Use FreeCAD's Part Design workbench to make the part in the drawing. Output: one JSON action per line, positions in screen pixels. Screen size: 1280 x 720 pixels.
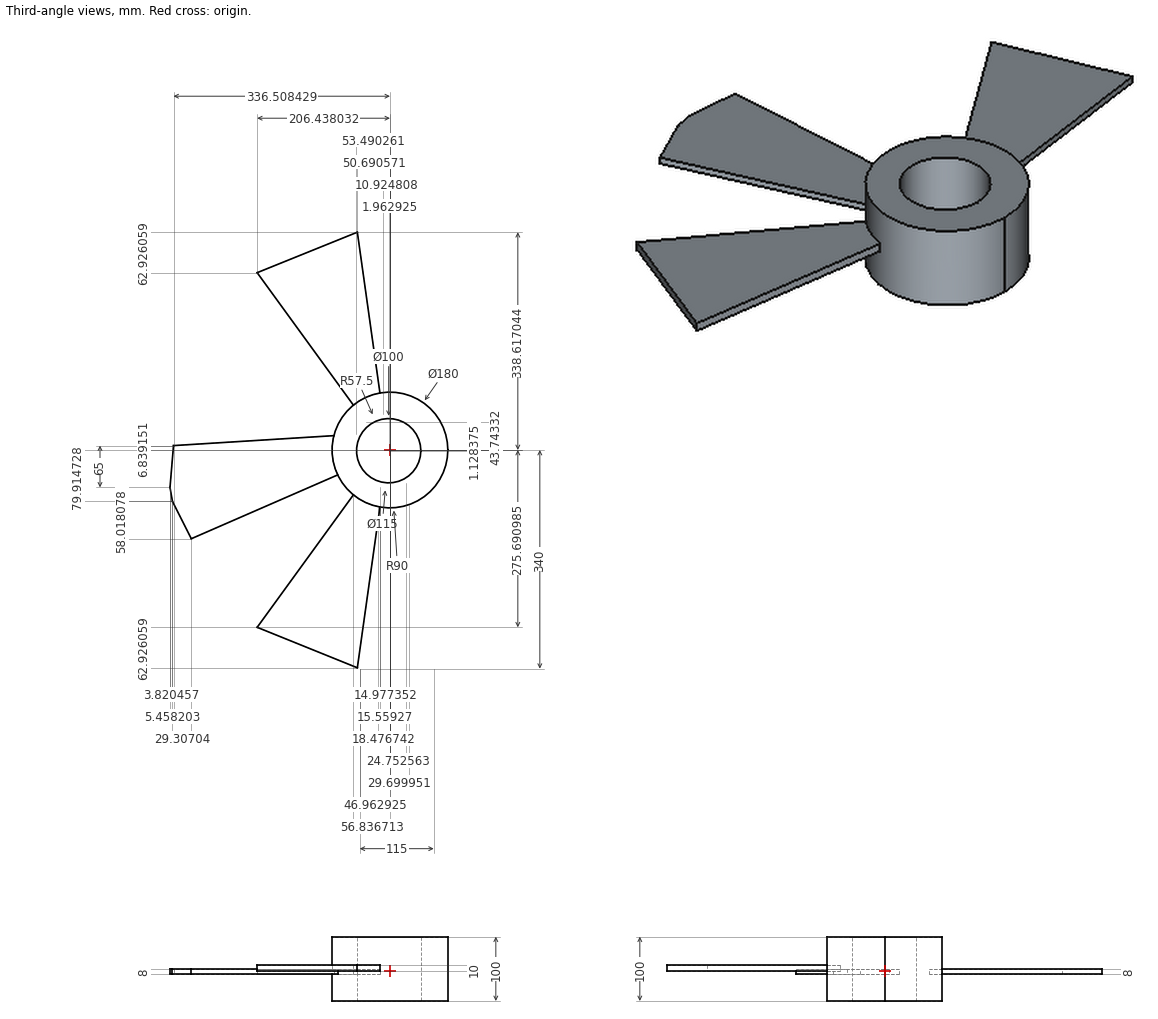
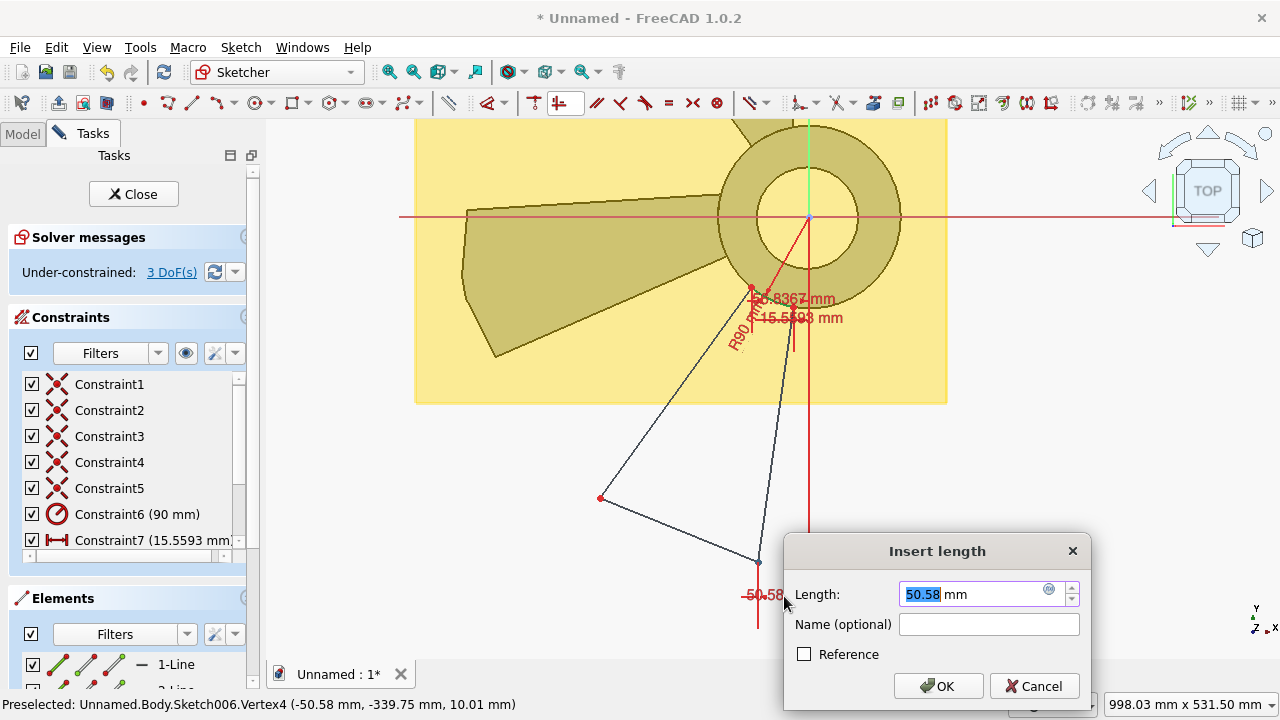
{"action": "type", "text": "50.690571"}
{"action": "key", "text": "Return"}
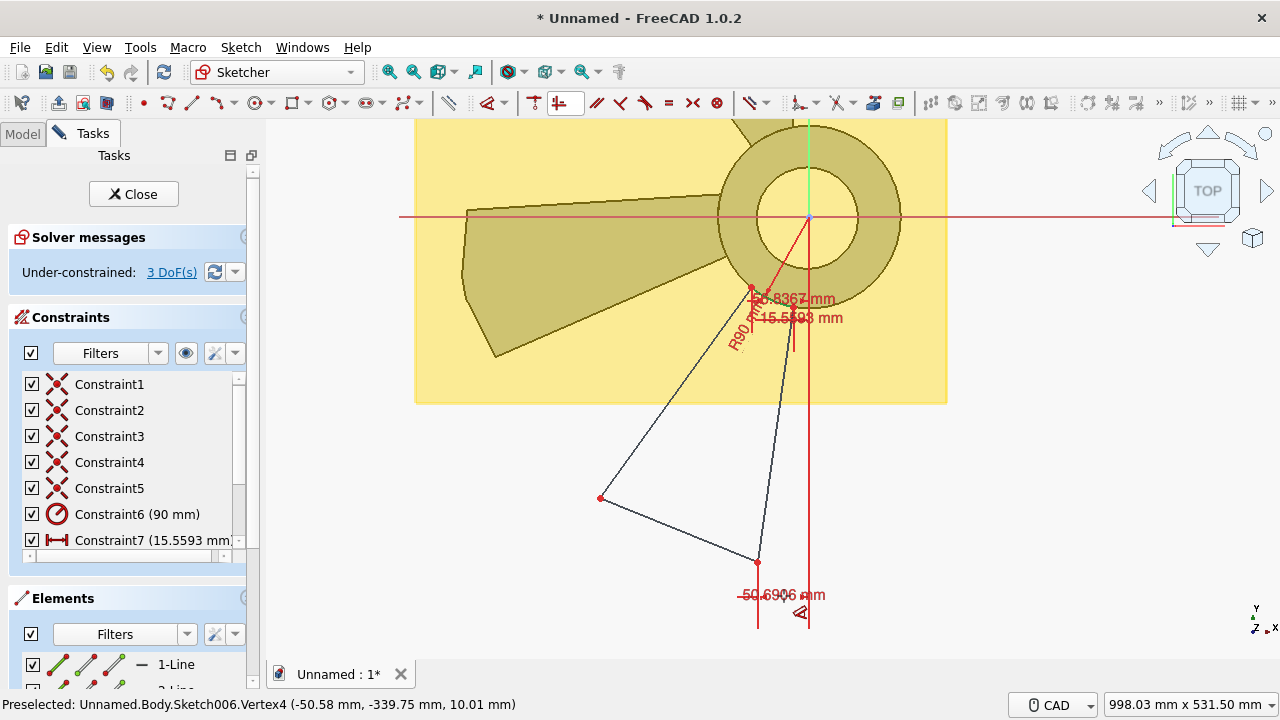
{"action": "left_click", "coordinate": [647, 517]}
{"action": "left_click", "coordinate": [566, 530]}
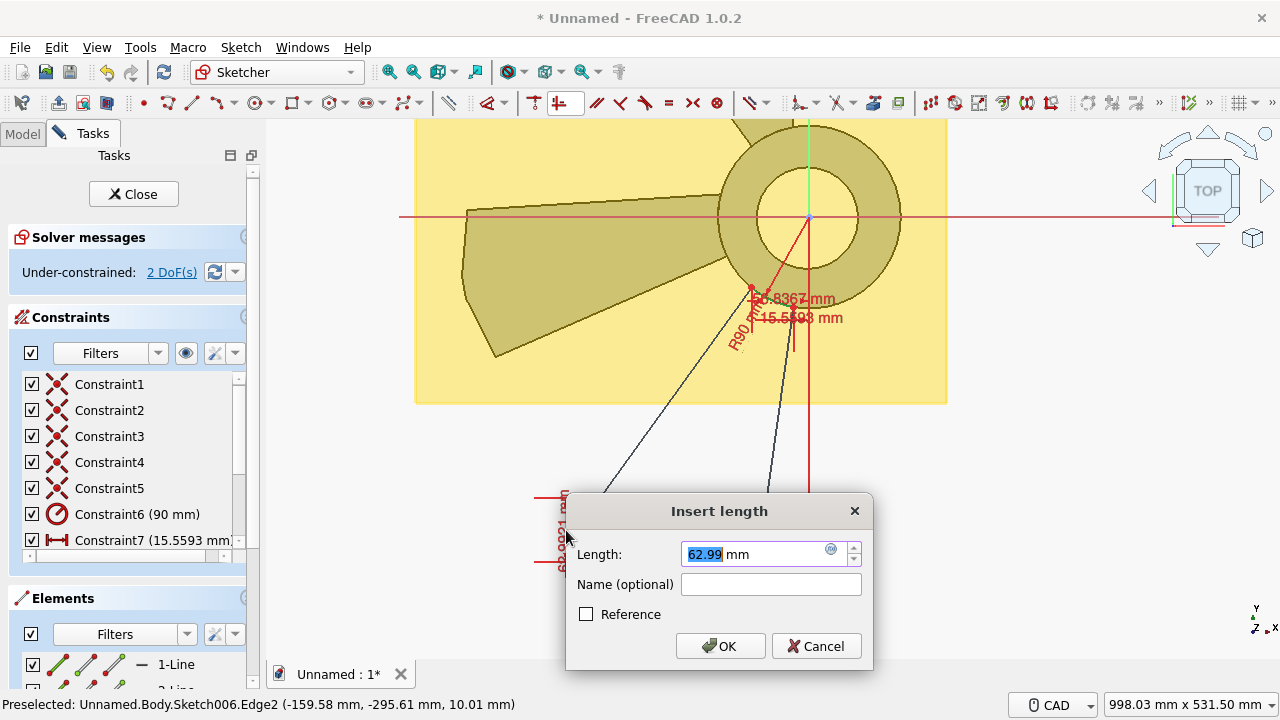
{"action": "type", "text": "62.926059"}
{"action": "key", "text": "Return"}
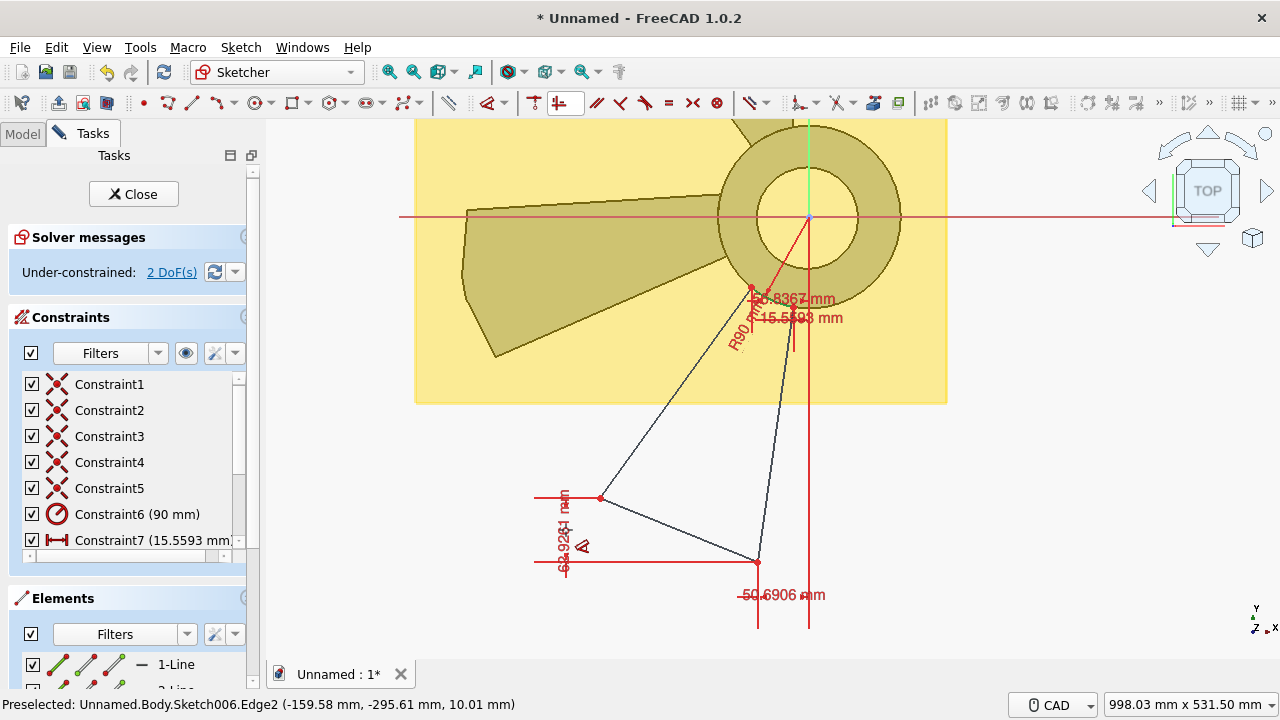
{"action": "left_click", "coordinate": [600, 498]}
{"action": "left_click", "coordinate": [705, 183]}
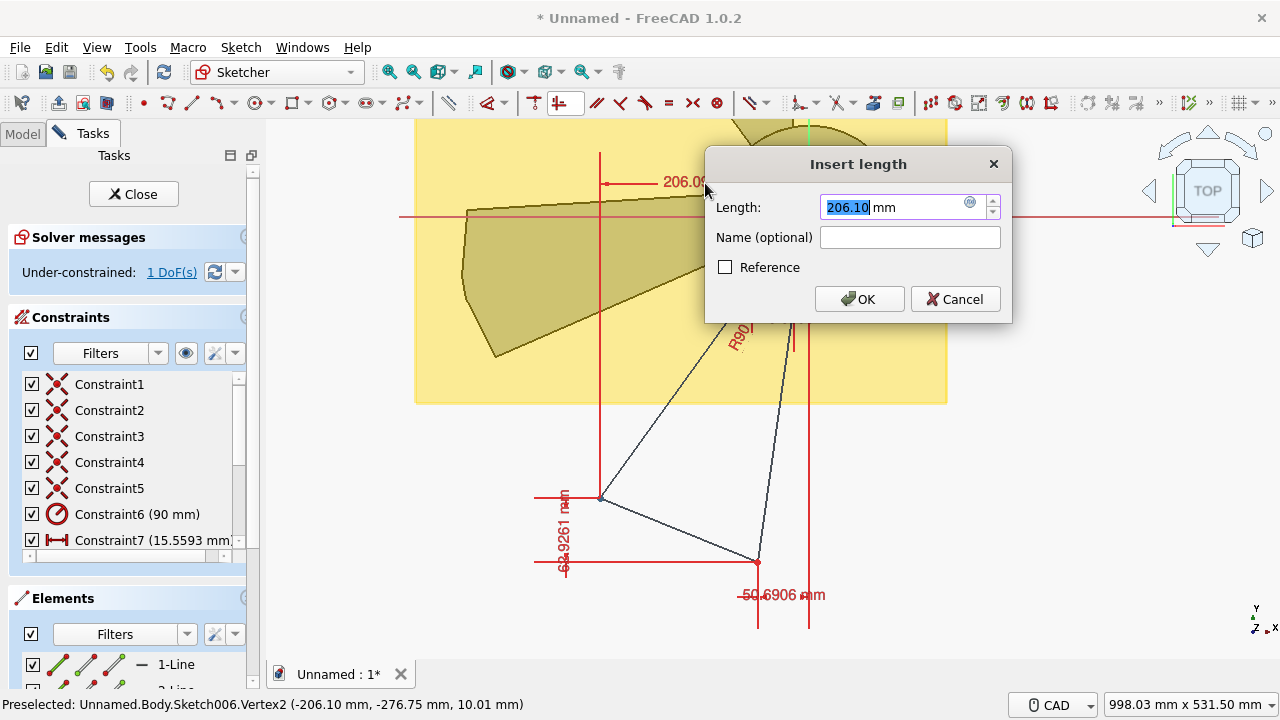
{"action": "type", "text": "206.438032"}
{"action": "key", "text": "Return"}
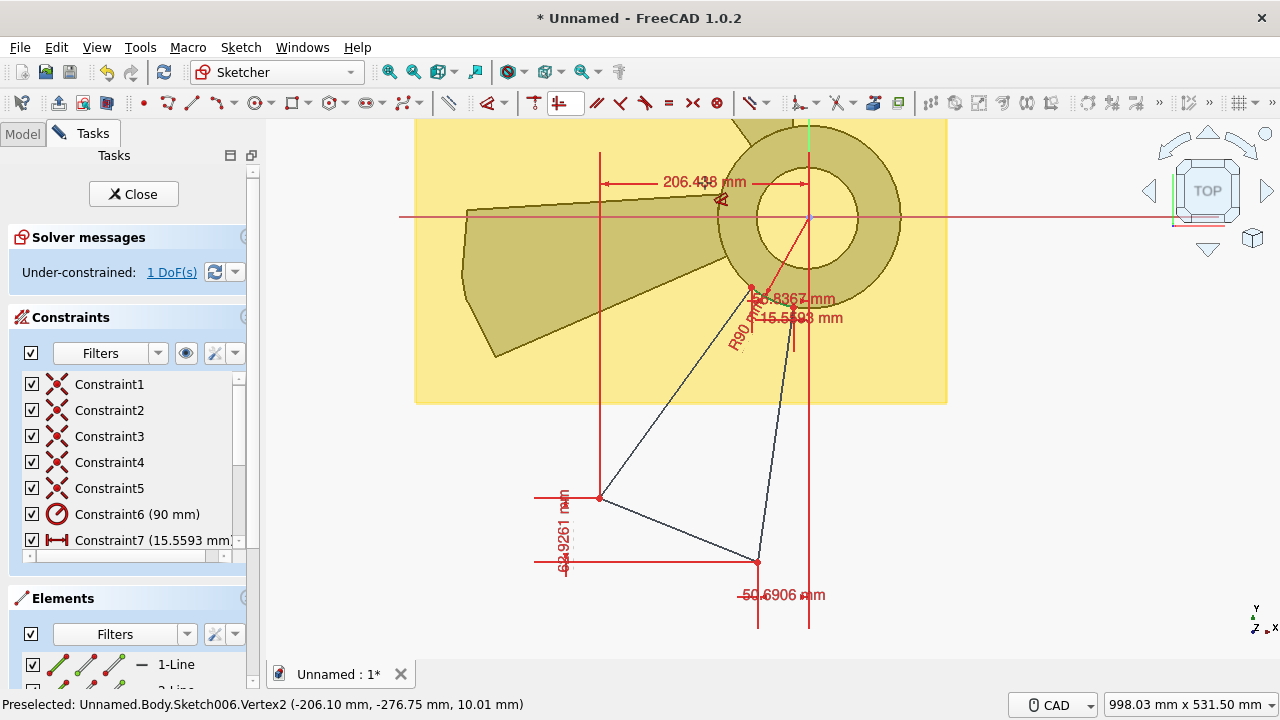
{"action": "left_click", "coordinate": [600, 498]}
{"action": "left_click", "coordinate": [566, 358]}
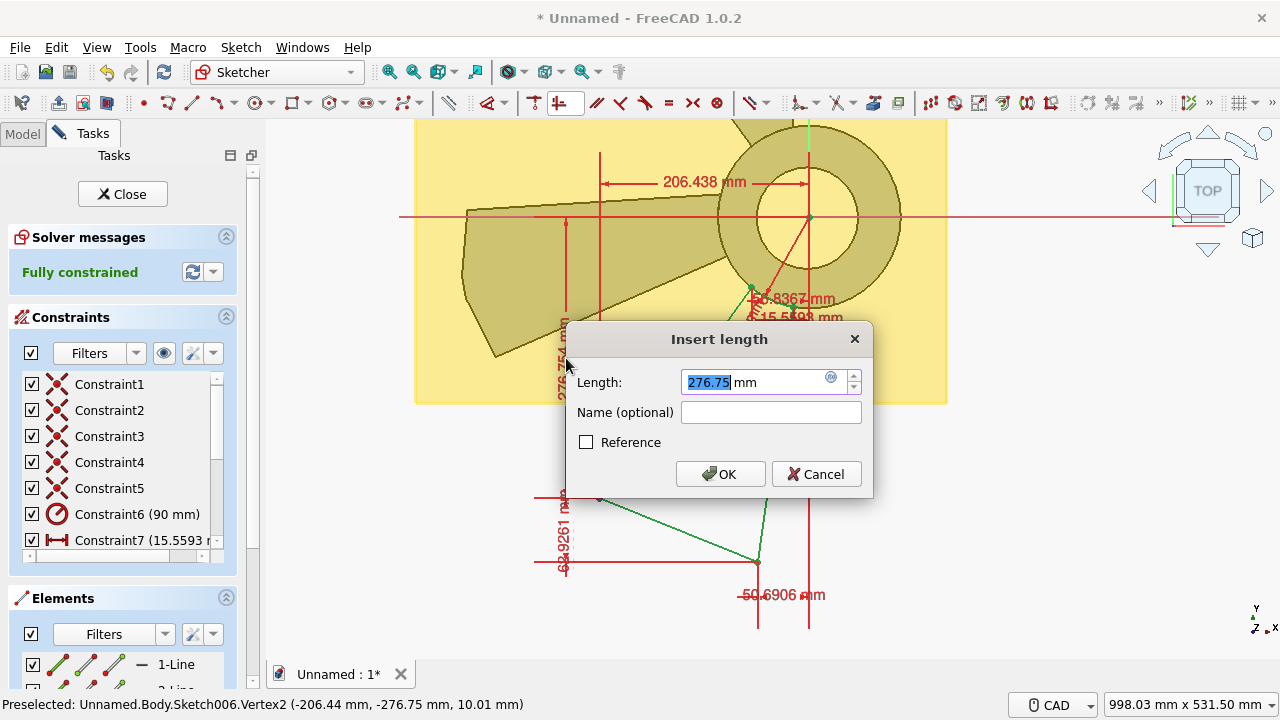
{"action": "type", "text": "275.690985"}
{"action": "key", "text": "Return"}
{"action": "key", "text": "Escape"}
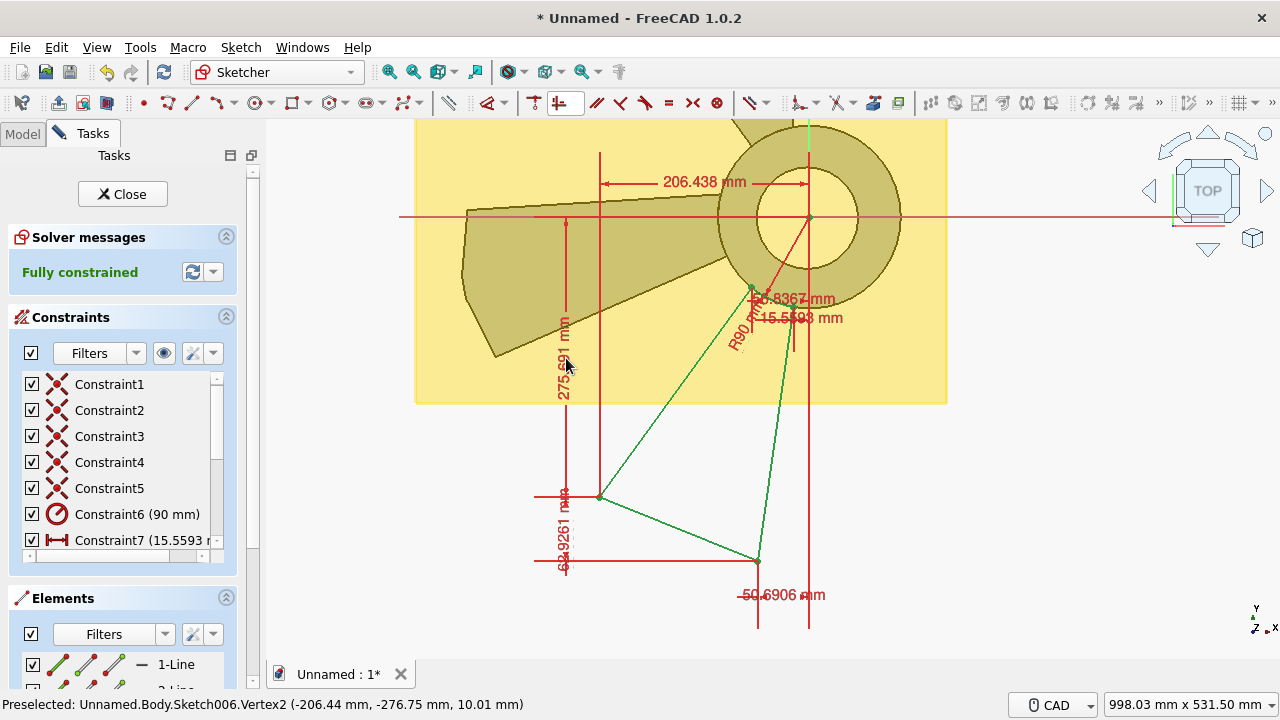
{"action": "left_click", "coordinate": [123, 194]}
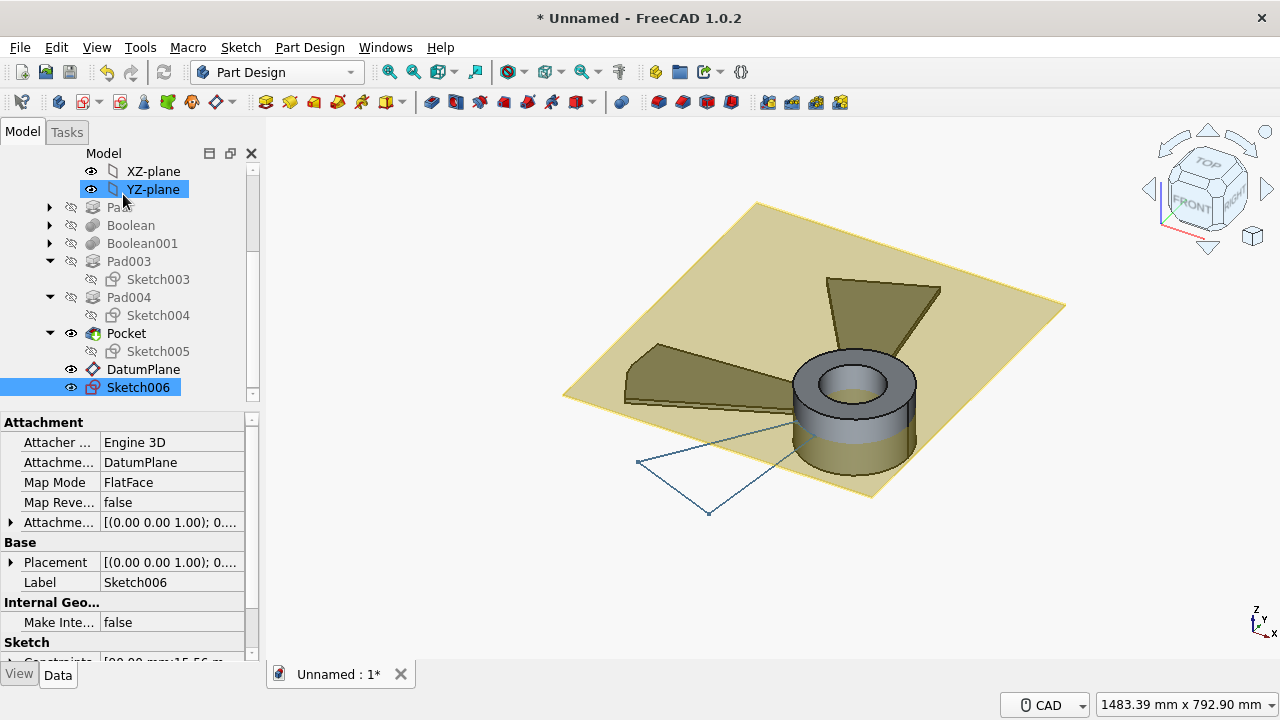
{"action": "left_click", "coordinate": [266, 102]}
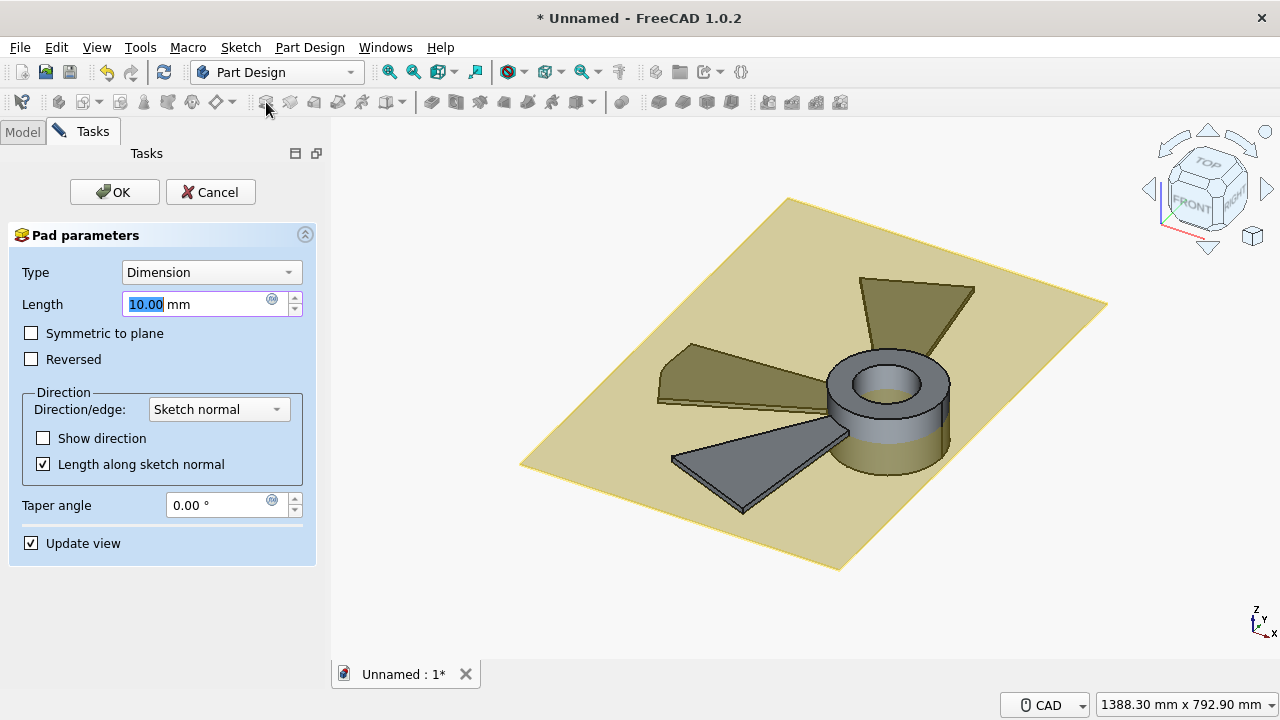
{"action": "type", "text": "10"}
{"action": "key", "text": "Tab"}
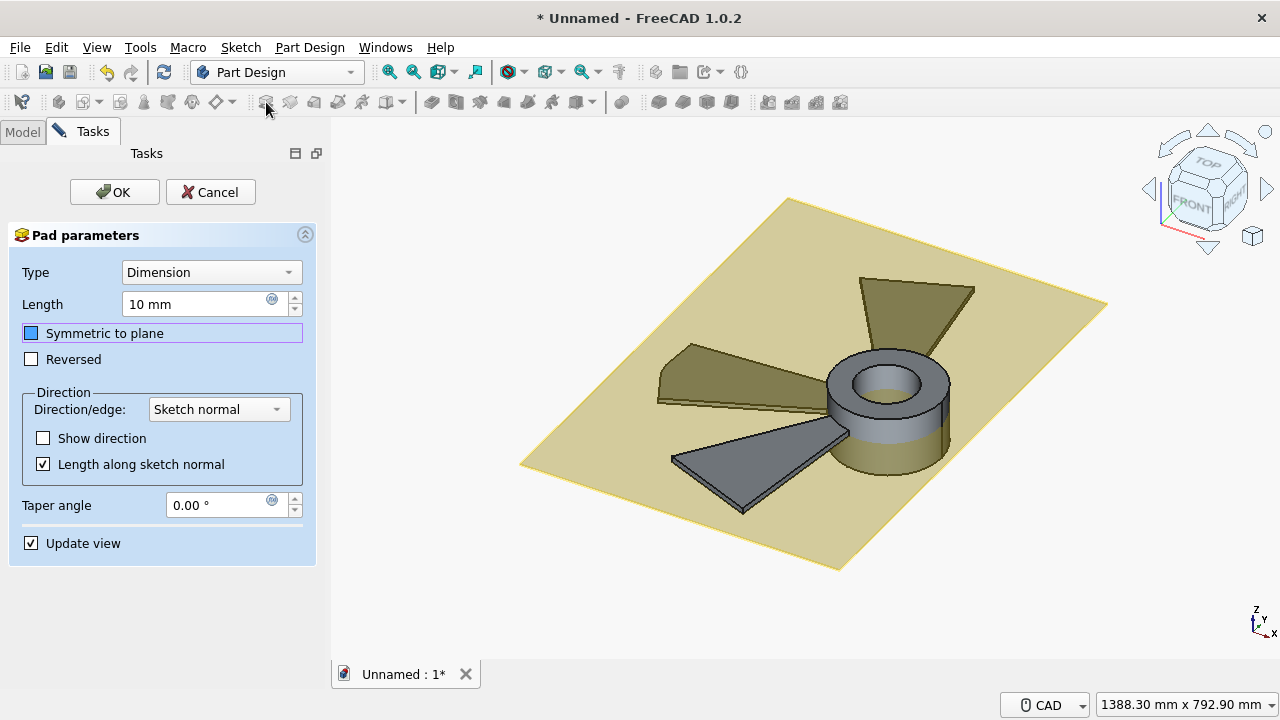
{"action": "left_click", "coordinate": [30, 359]}